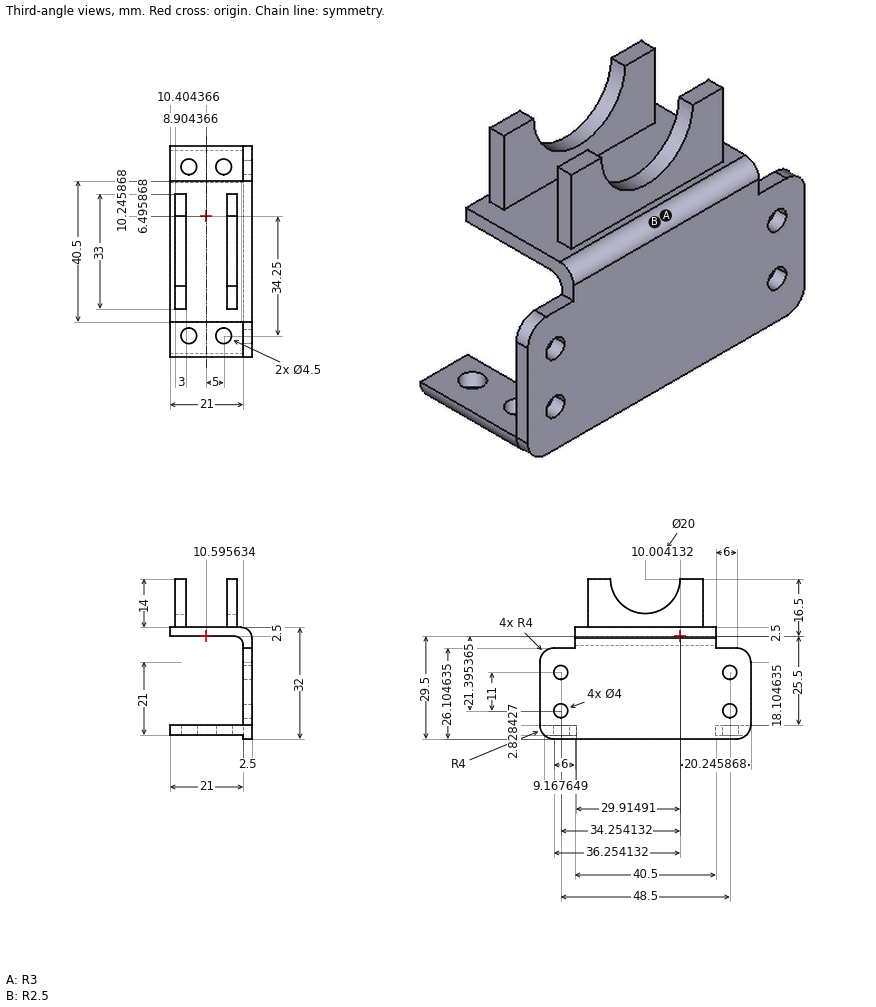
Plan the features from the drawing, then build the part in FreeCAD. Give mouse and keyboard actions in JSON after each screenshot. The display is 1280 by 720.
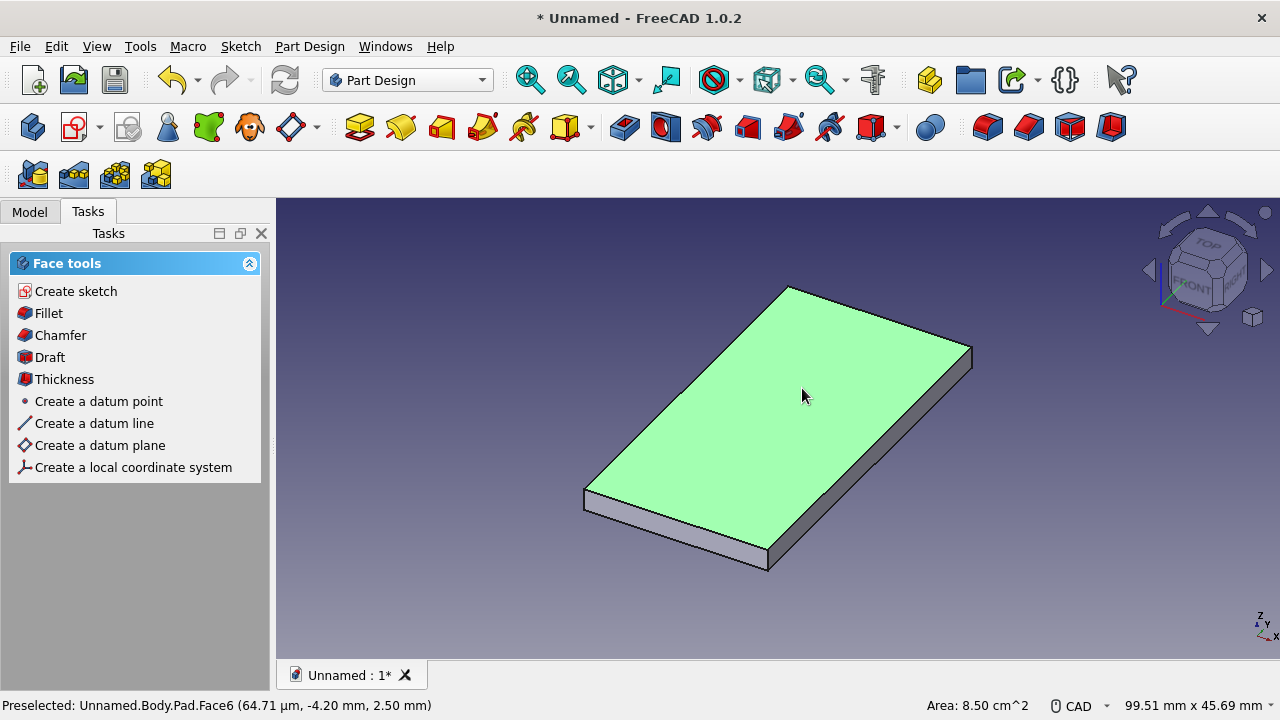
{"action": "left_click", "coordinate": [74, 128]}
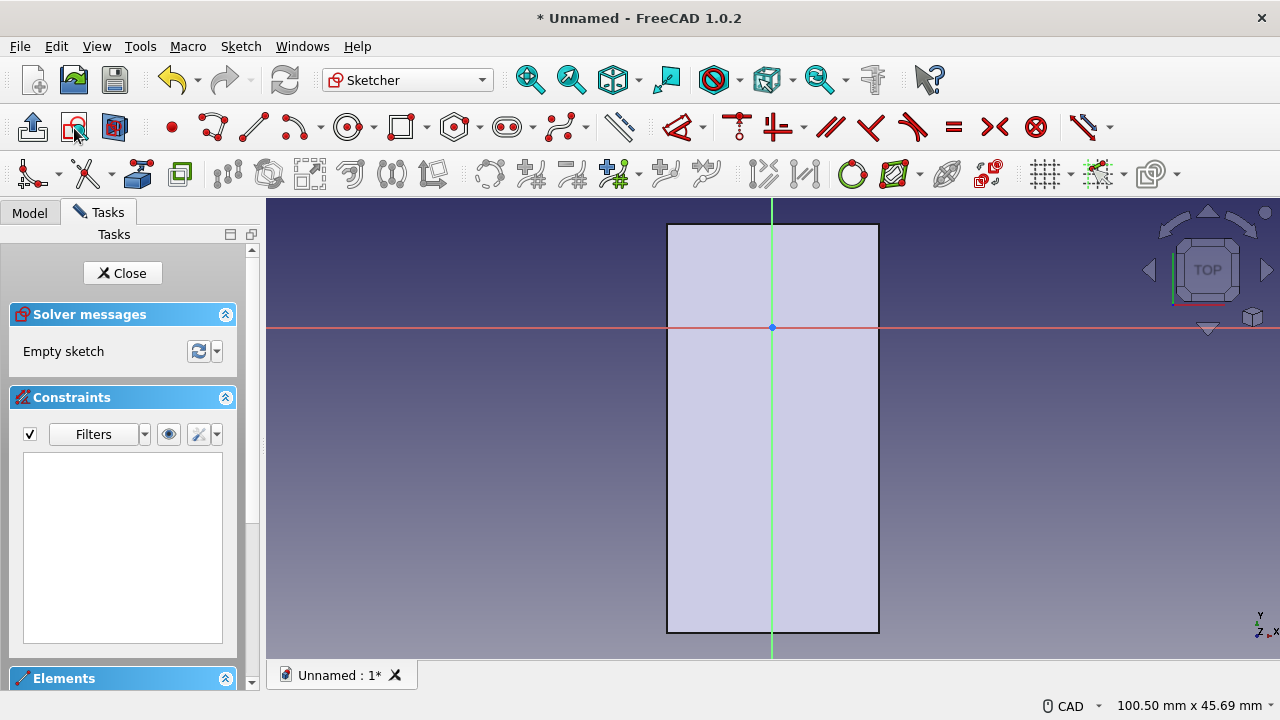
{"action": "left_click", "coordinate": [400, 128]}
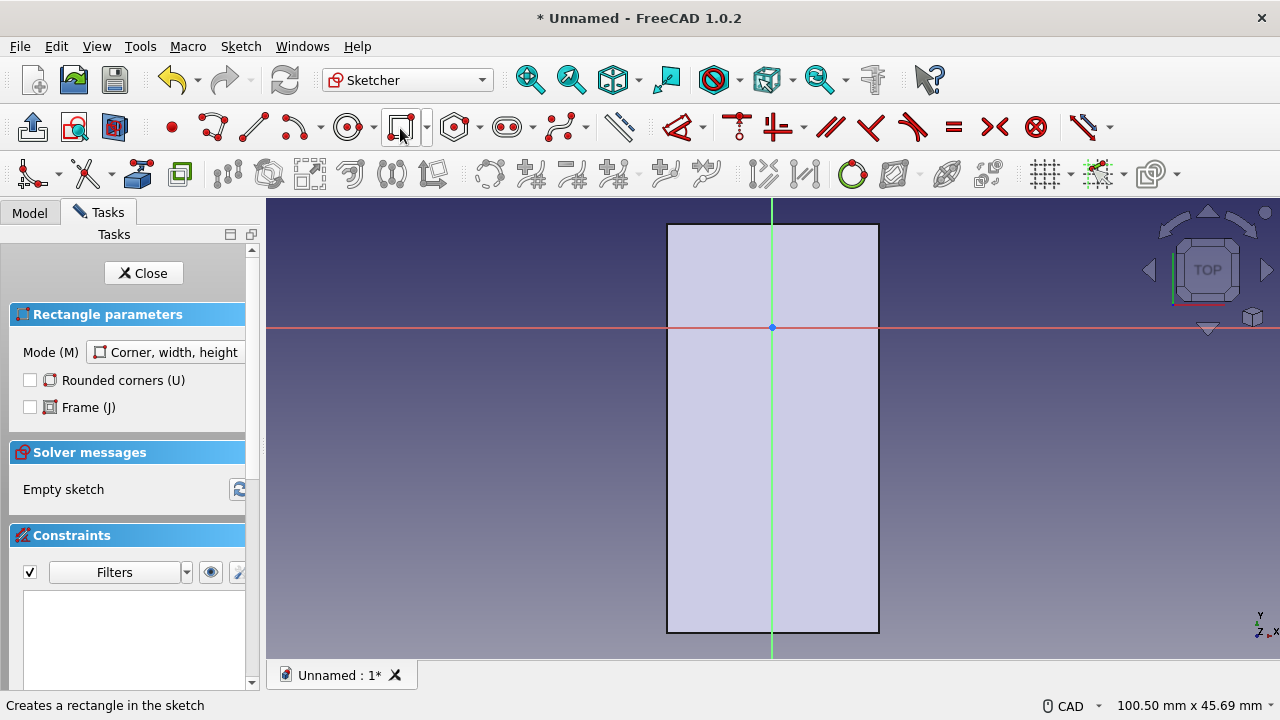
{"action": "left_click", "coordinate": [682, 262]}
{"action": "left_click", "coordinate": [712, 595]}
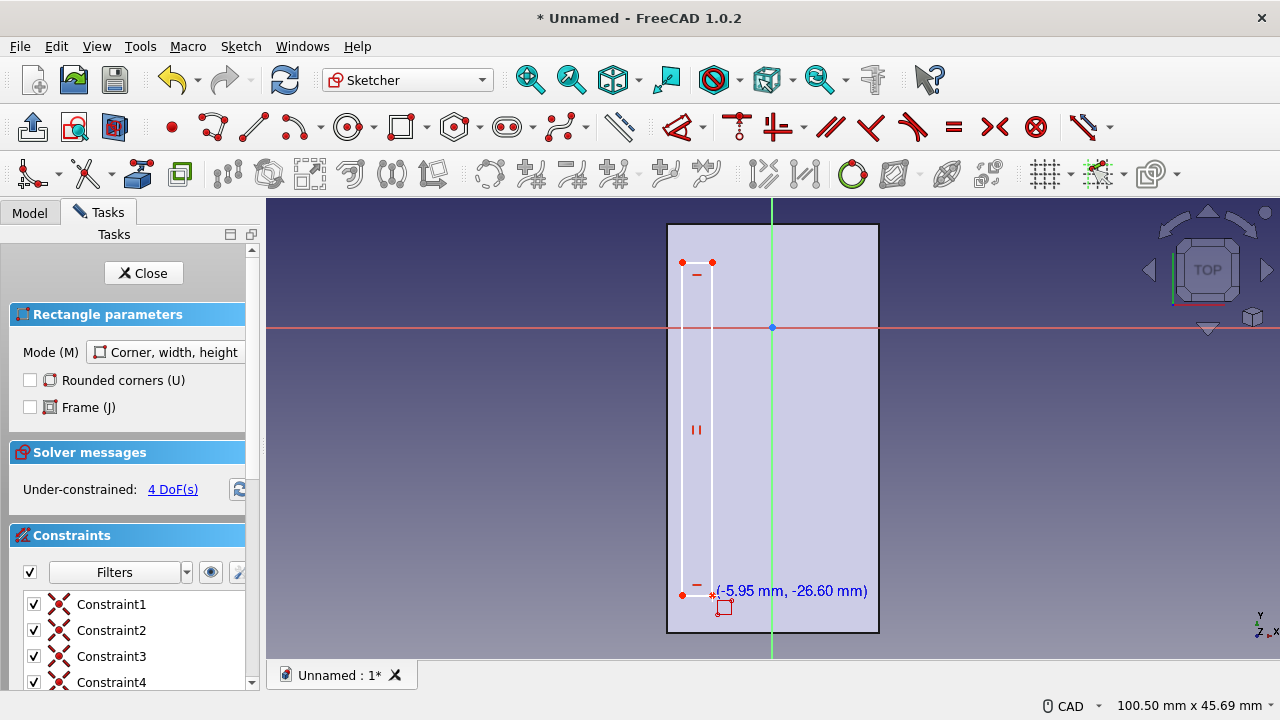
{"action": "left_click", "coordinate": [832, 262]}
{"action": "left_click", "coordinate": [862, 595]}
{"action": "key", "text": "Escape"}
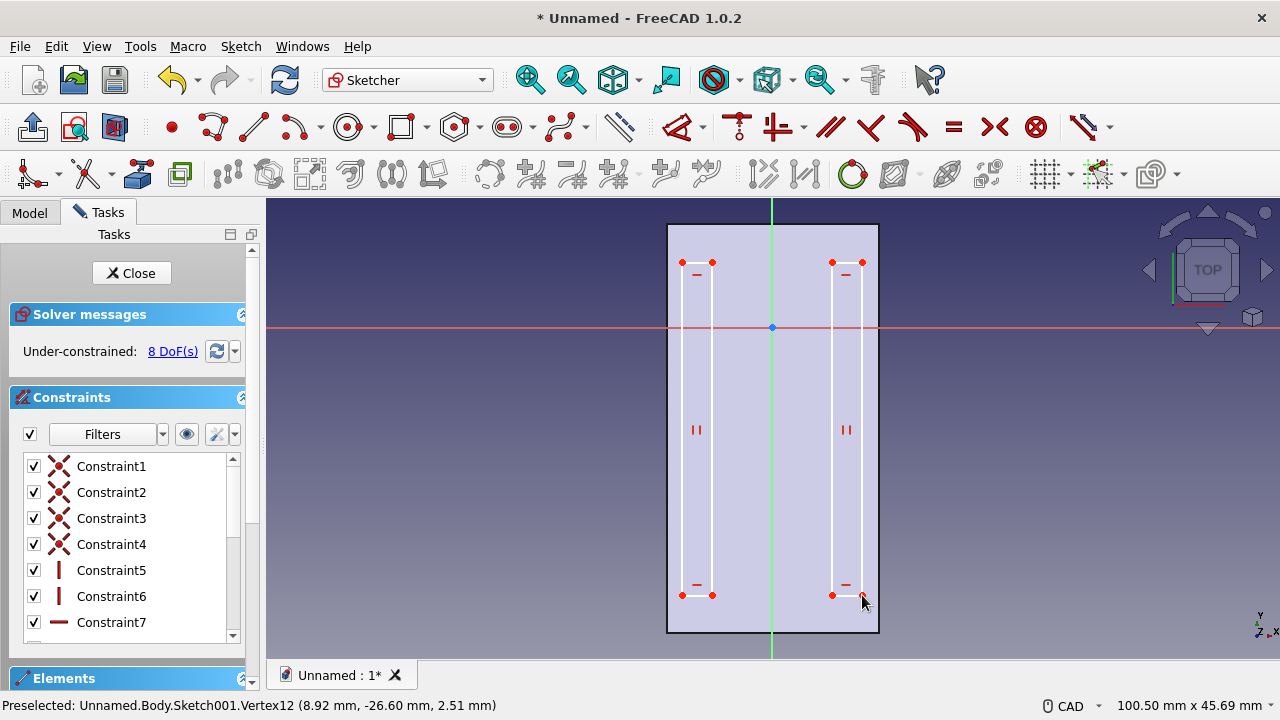
{"action": "left_click", "coordinate": [712, 263]}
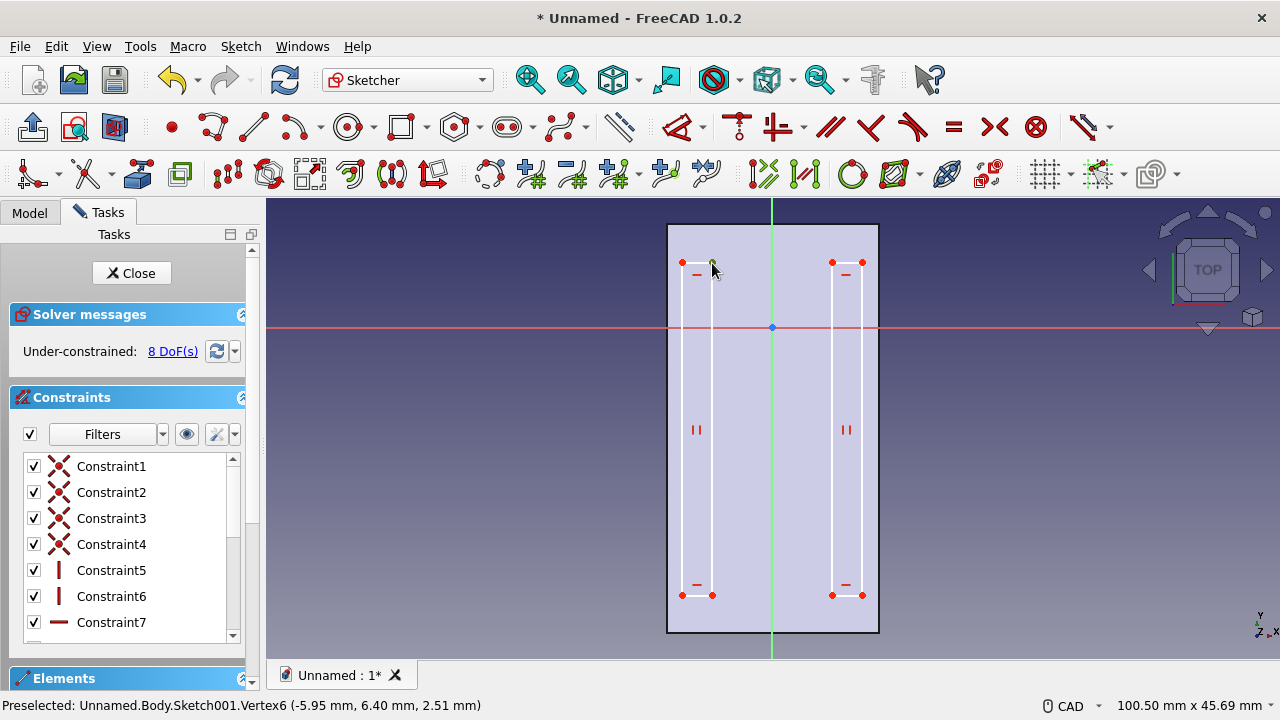
{"action": "left_click", "coordinate": [832, 263]}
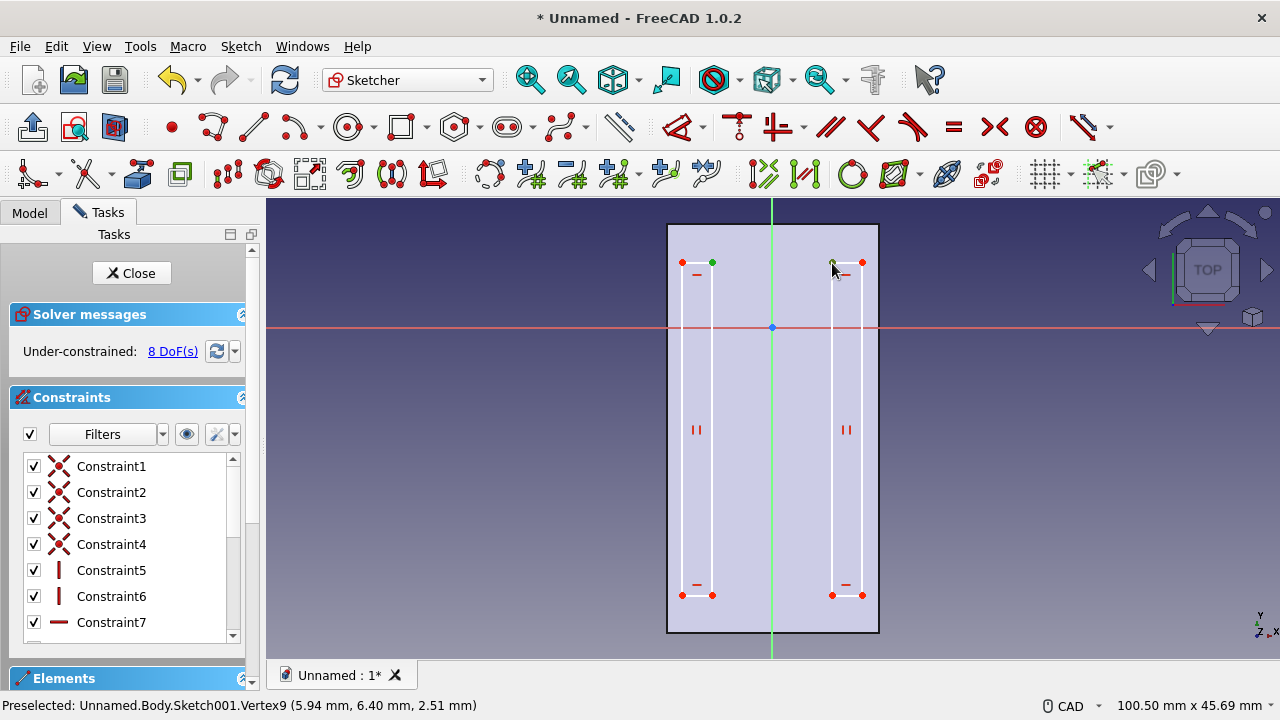
{"action": "left_click", "coordinate": [772, 602]}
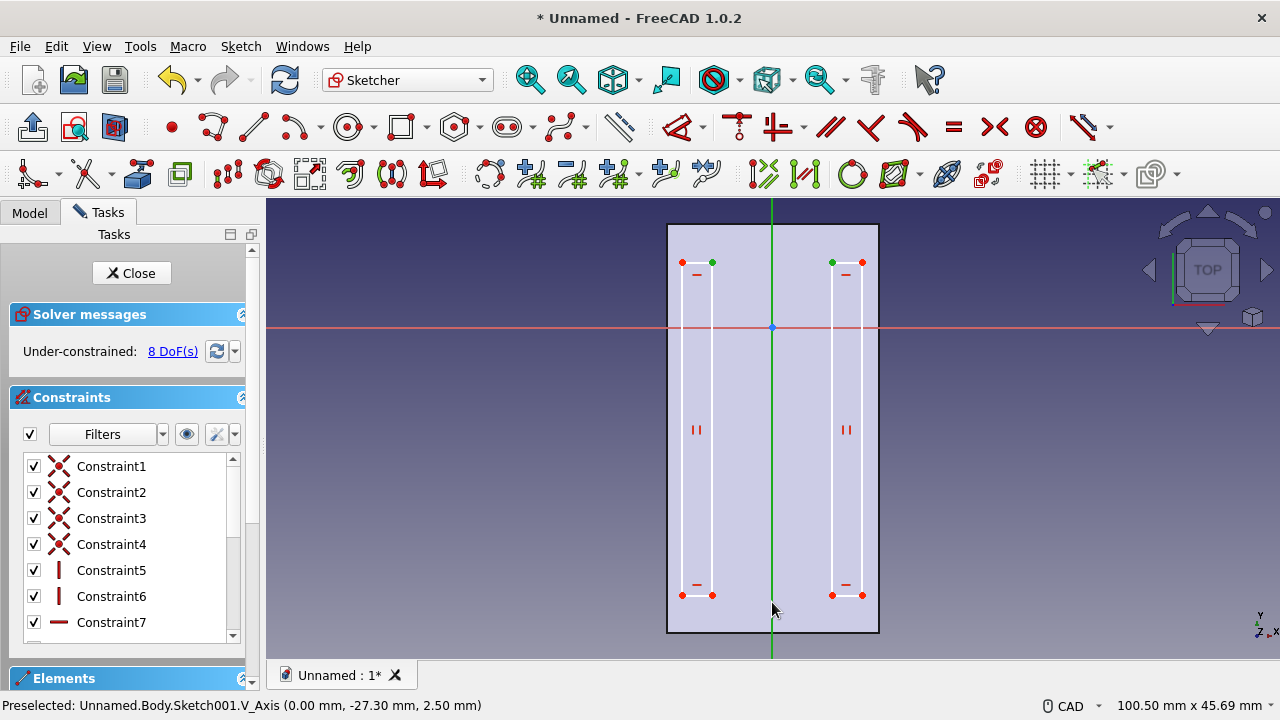
{"action": "left_click", "coordinate": [995, 128]}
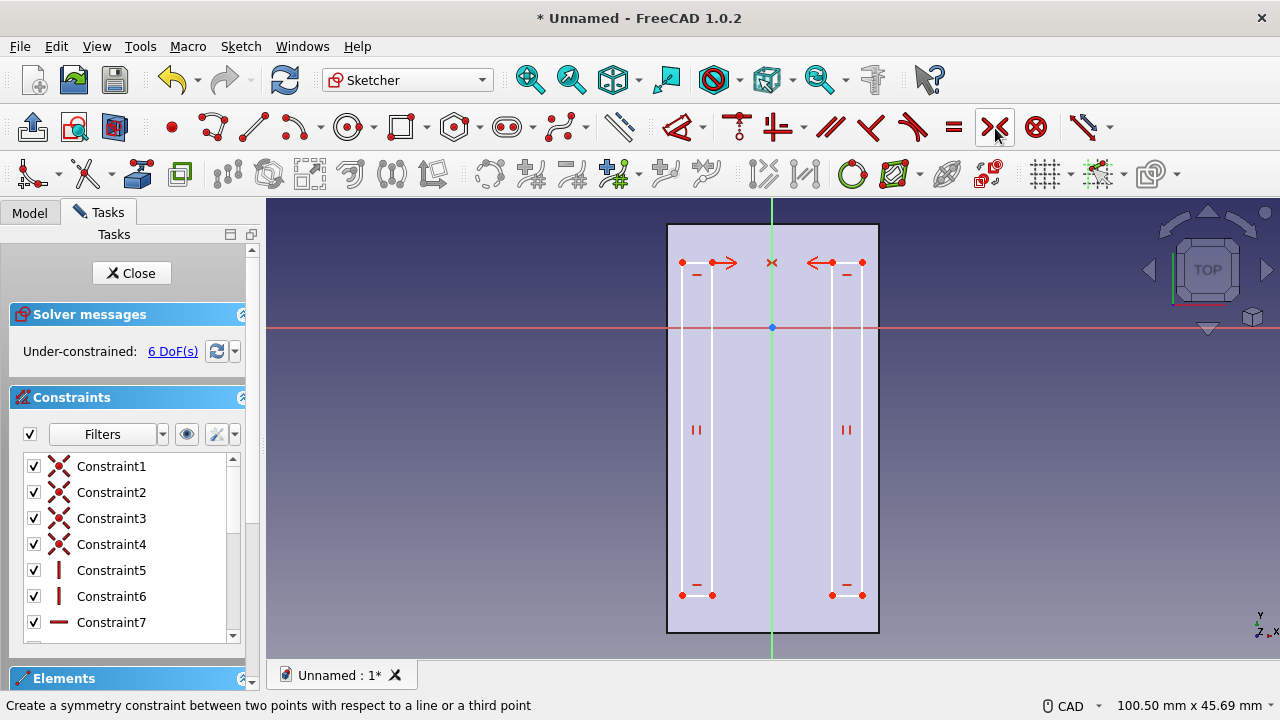
{"action": "left_click", "coordinate": [682, 596]}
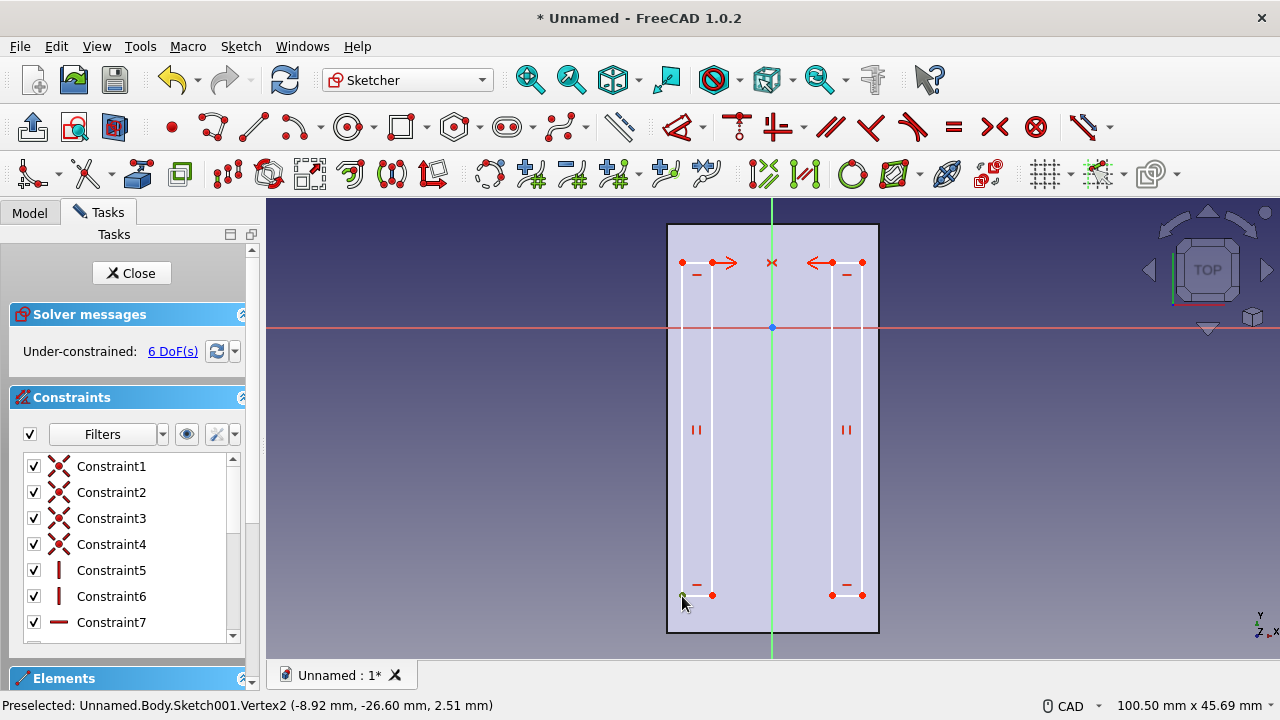
{"action": "left_click", "coordinate": [862, 596]}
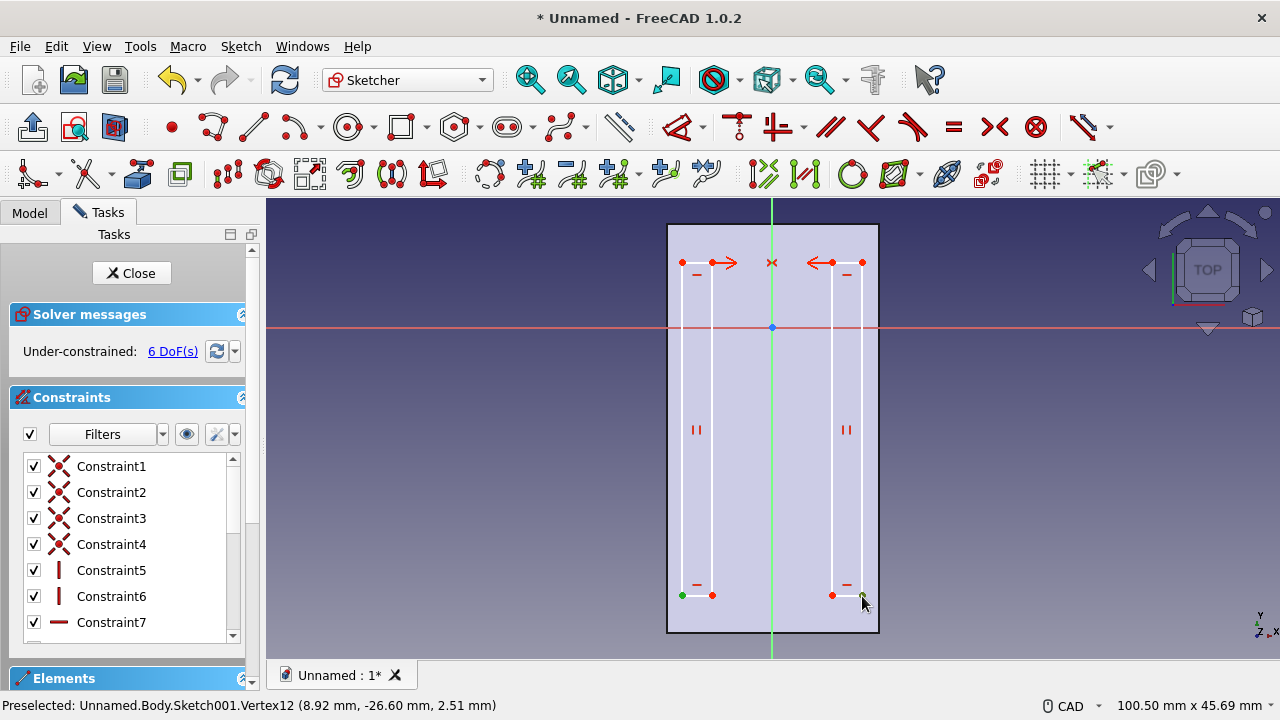
{"action": "left_click", "coordinate": [772, 602]}